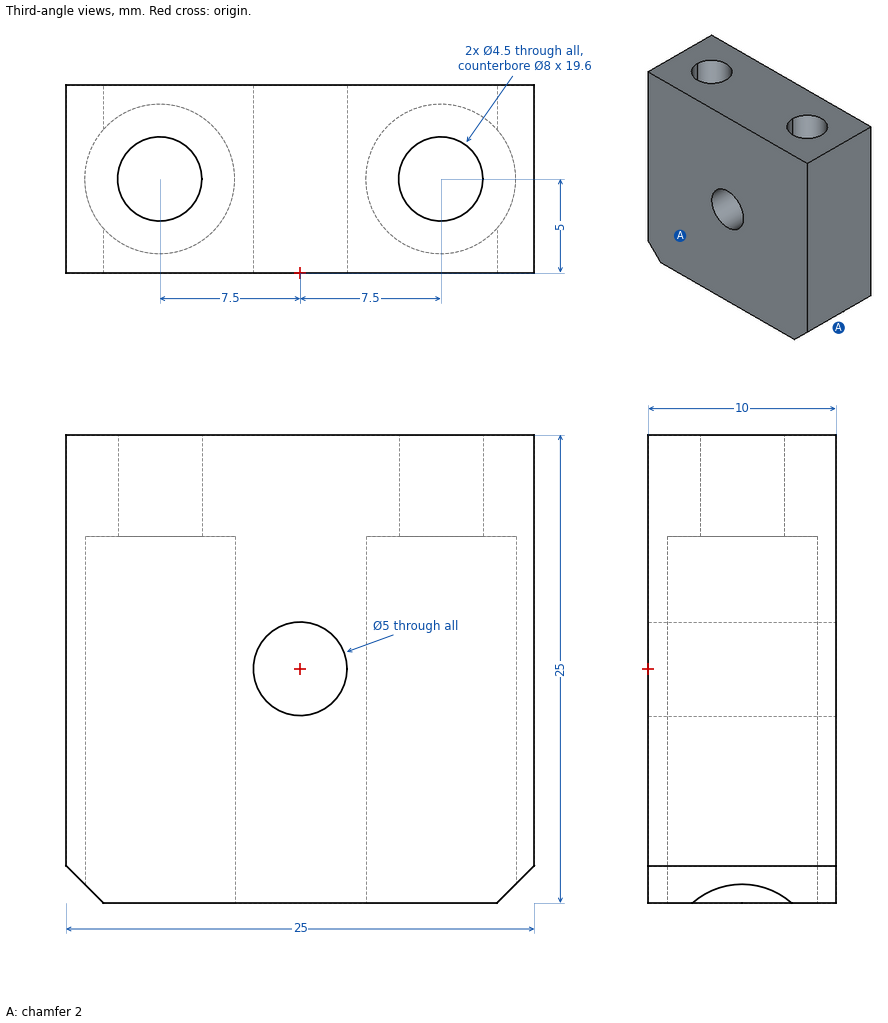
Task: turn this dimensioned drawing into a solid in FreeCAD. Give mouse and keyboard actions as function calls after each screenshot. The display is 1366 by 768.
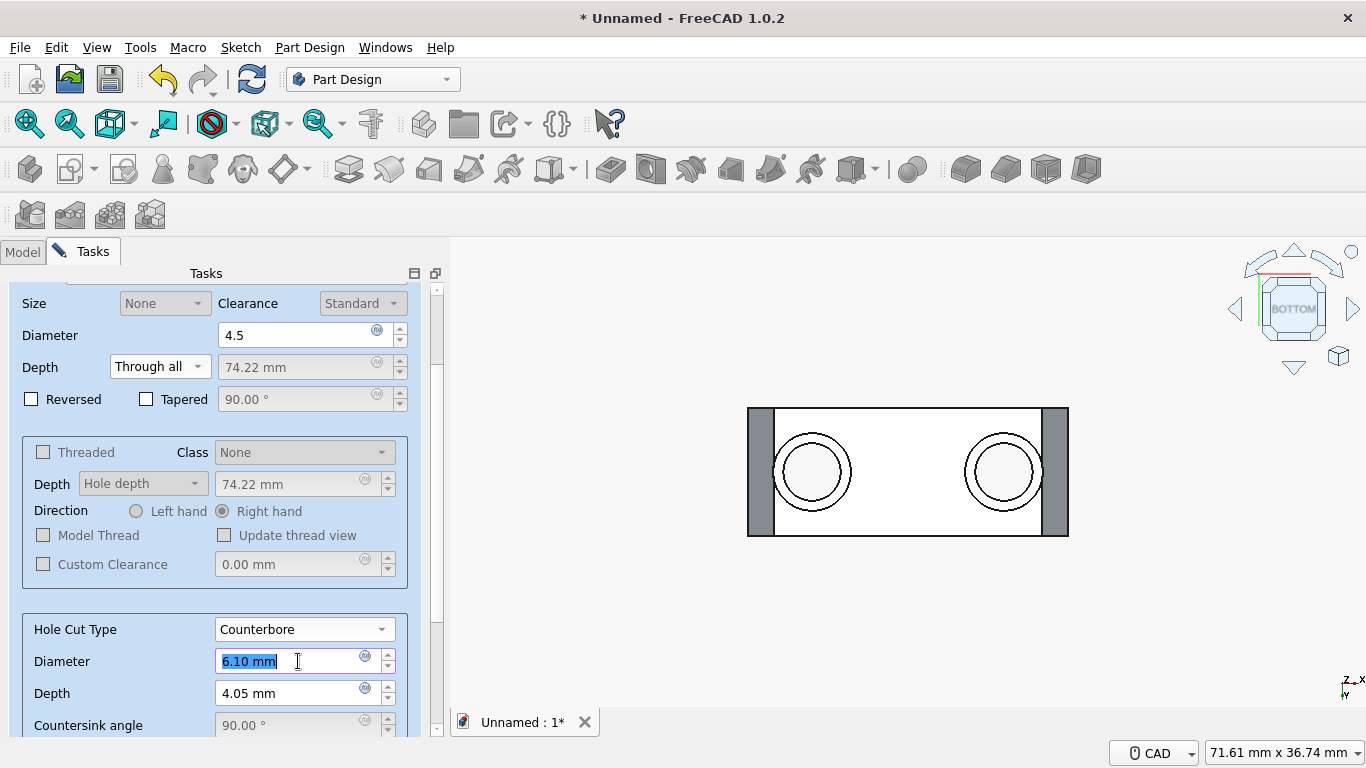
text(8)
key(Tab)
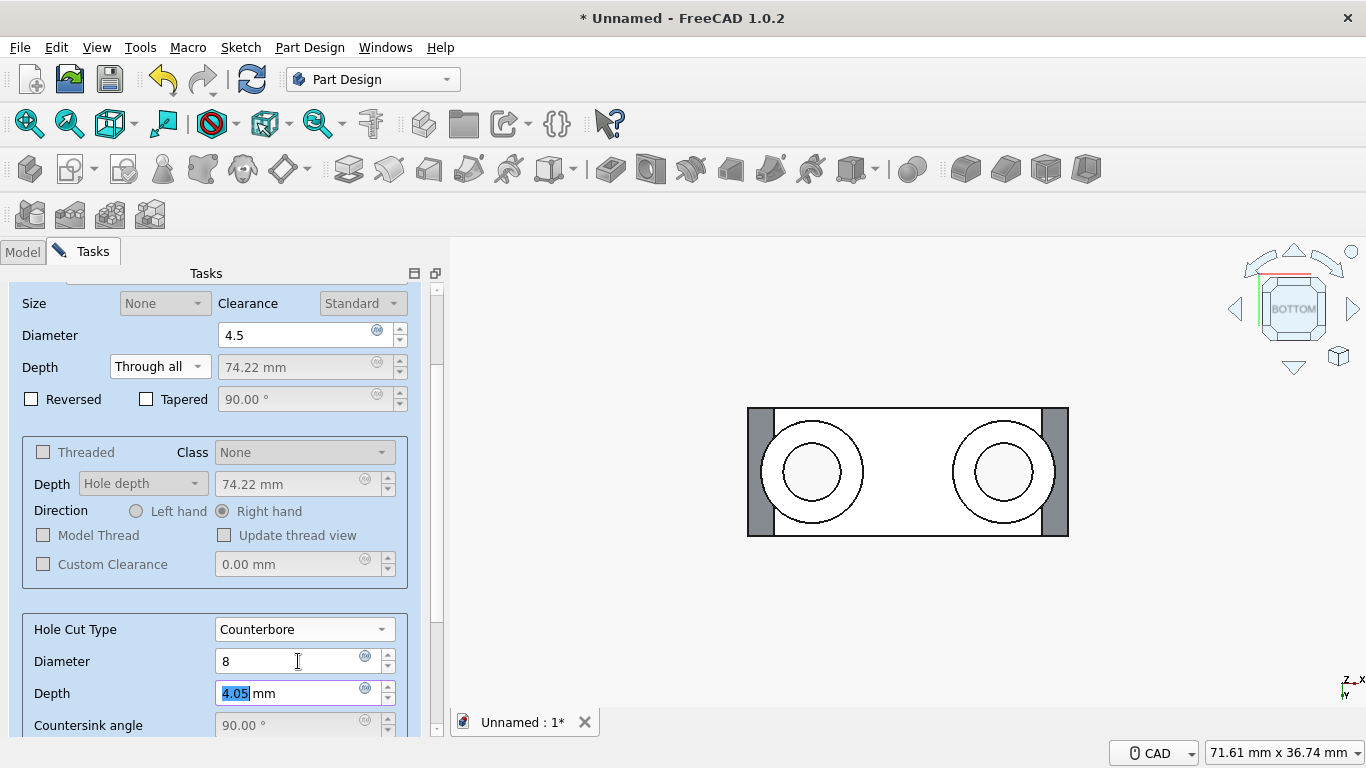
text(19.6)
key(Tab)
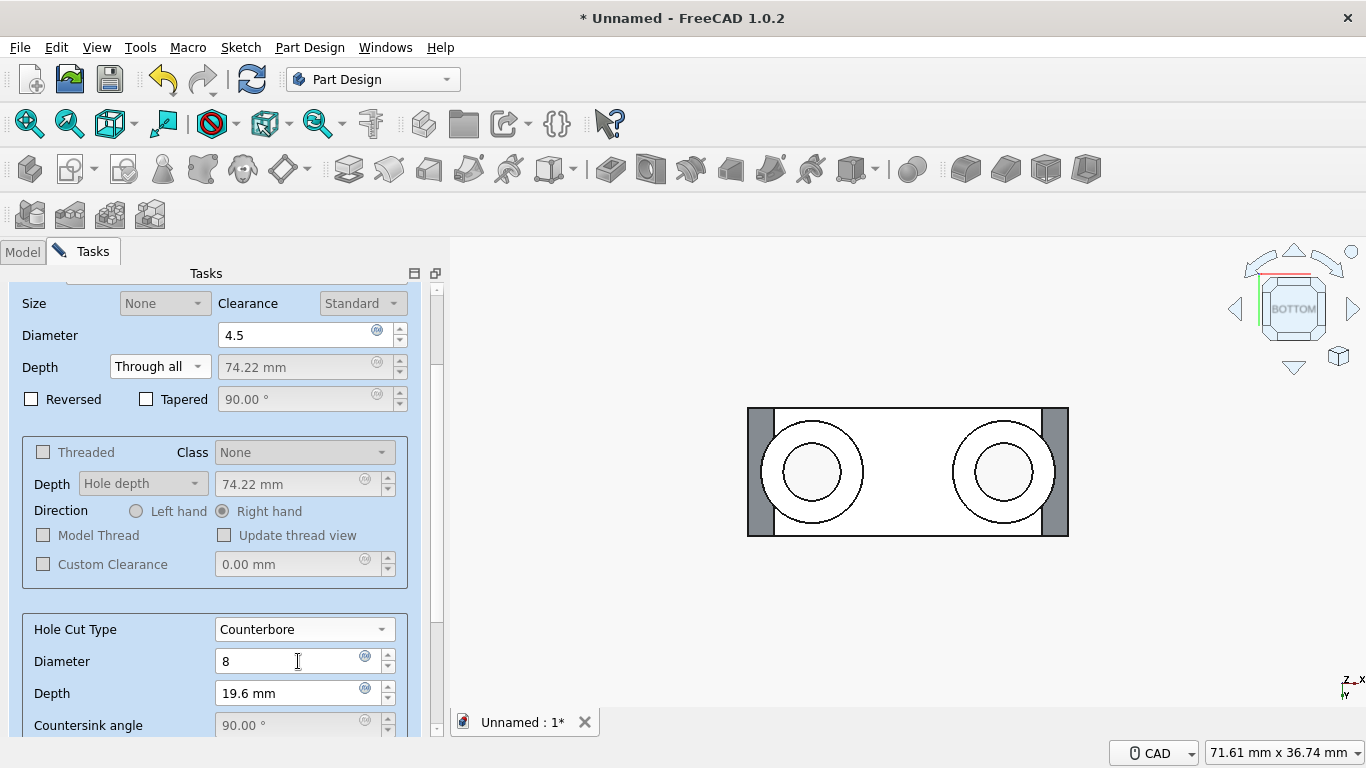
scroll(437, 510, up, 3)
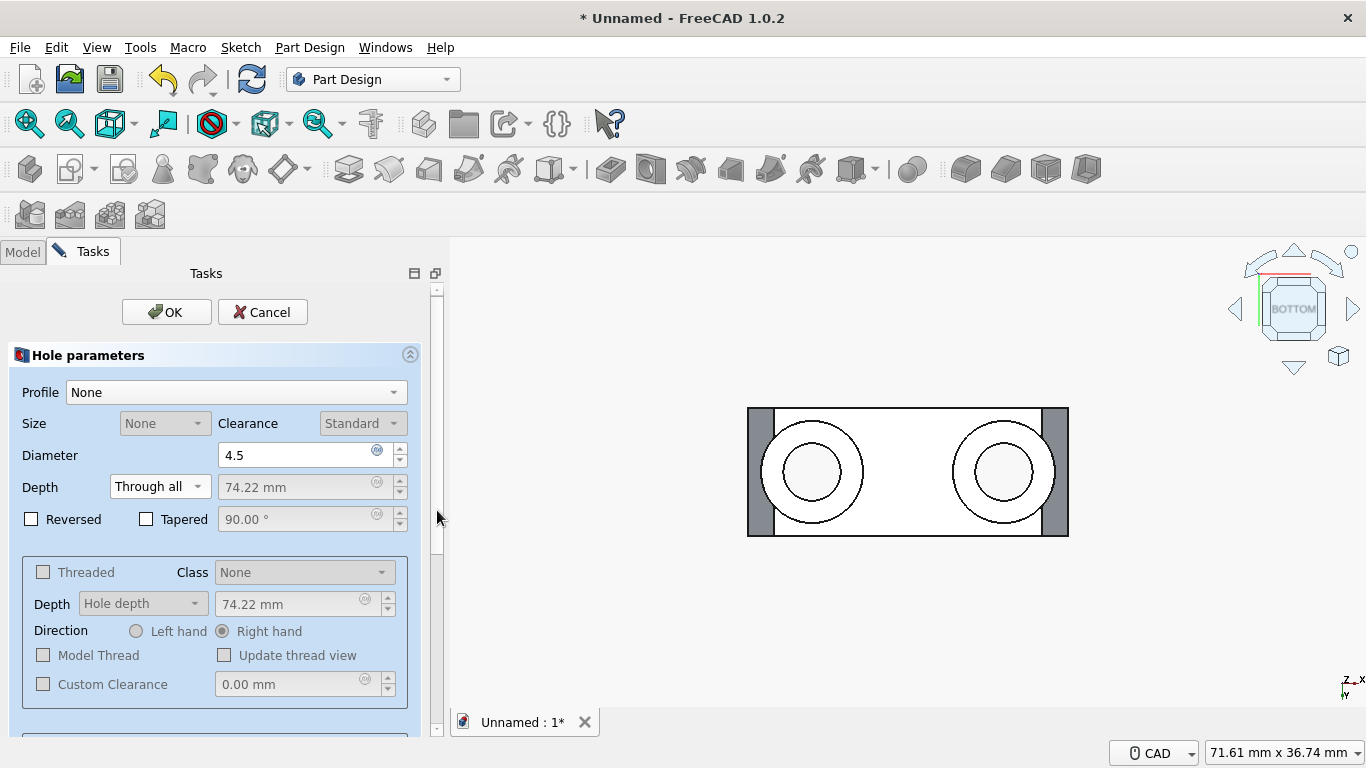
click(167, 312)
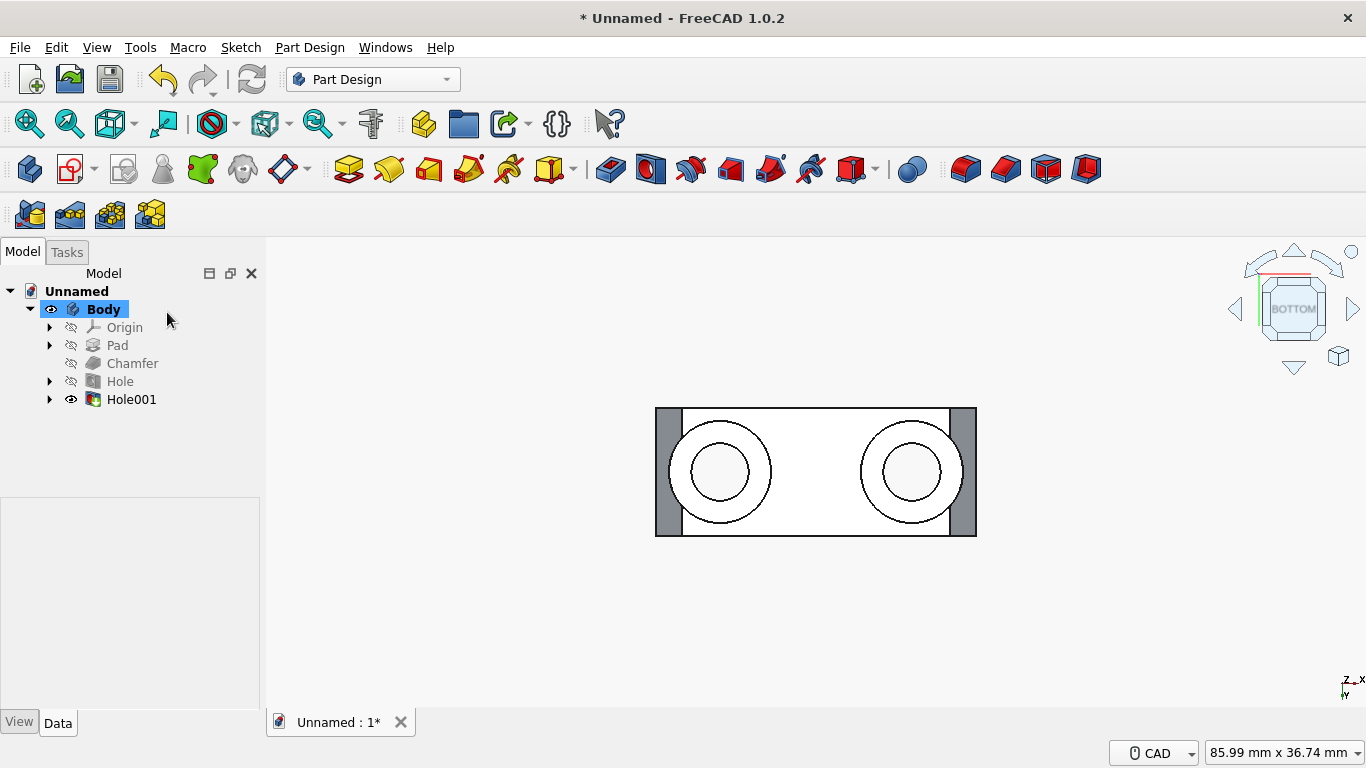
key(0)